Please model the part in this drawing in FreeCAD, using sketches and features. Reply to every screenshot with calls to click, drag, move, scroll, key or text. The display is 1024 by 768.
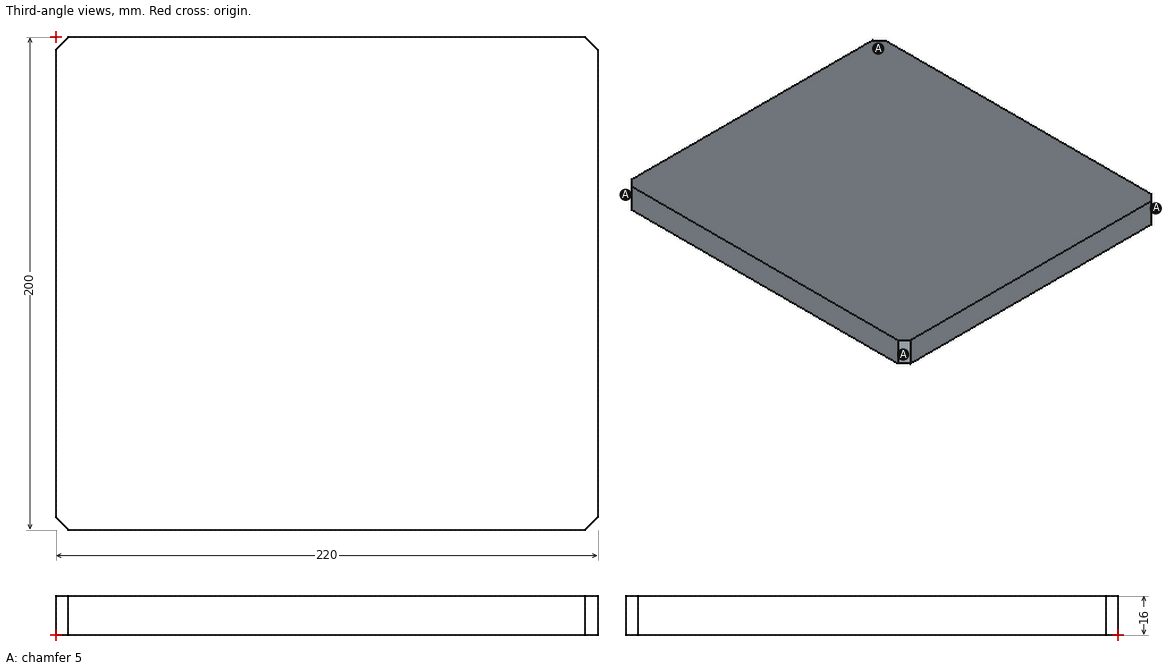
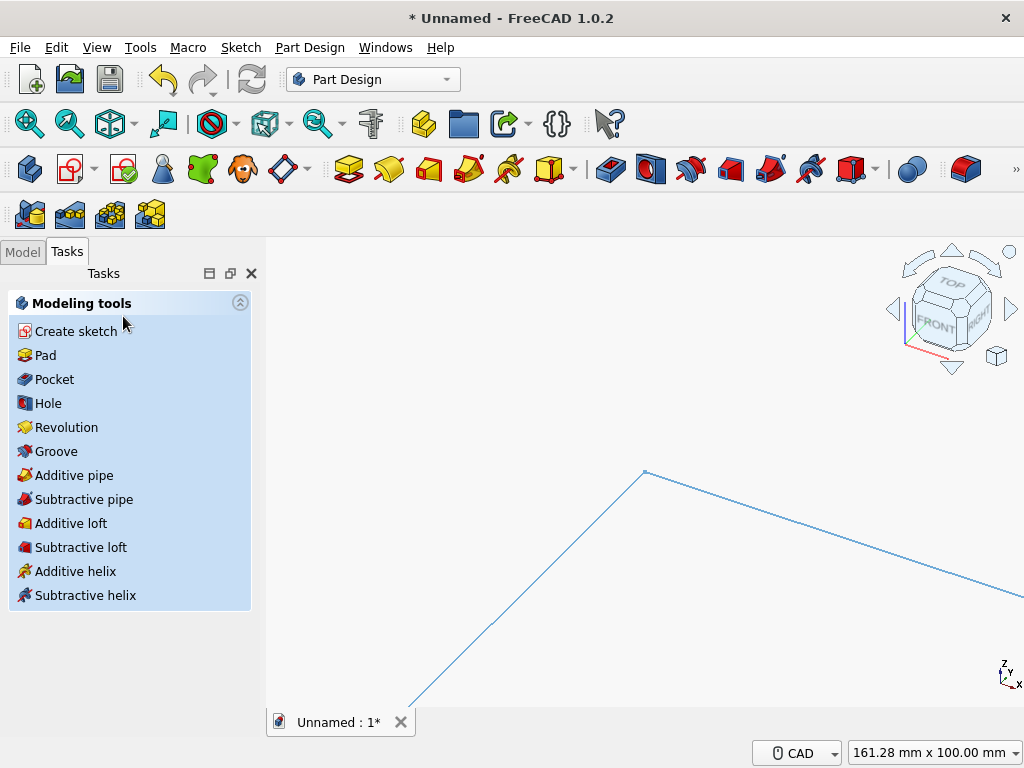
click(350, 170)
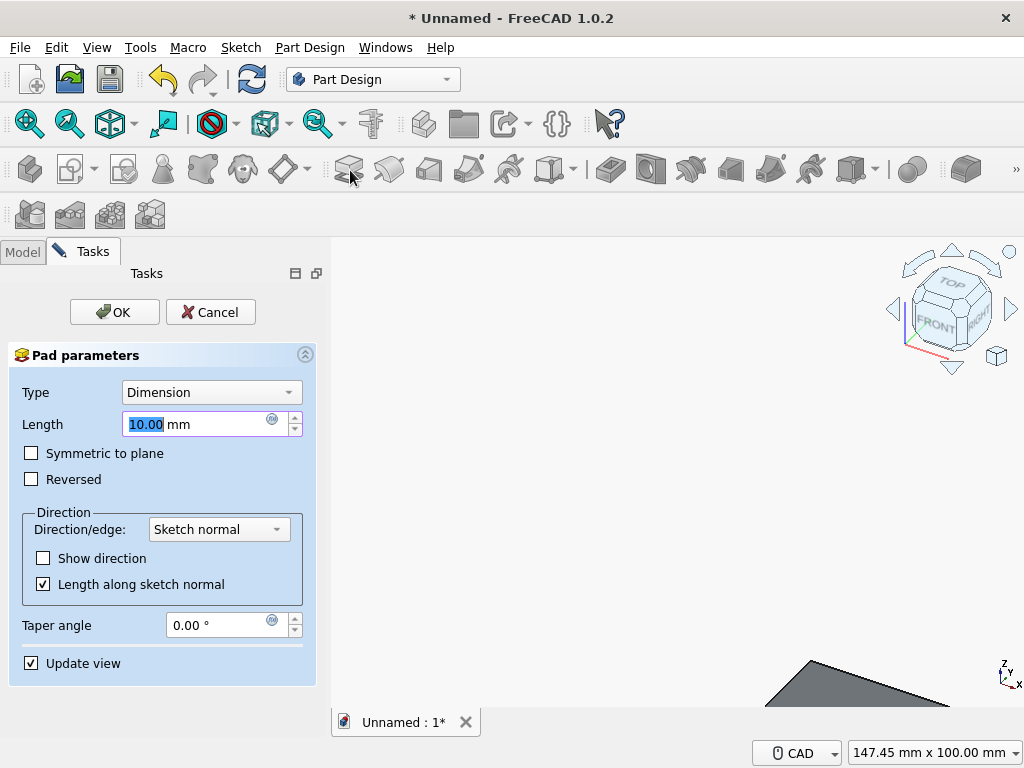
text(16)
key(Tab)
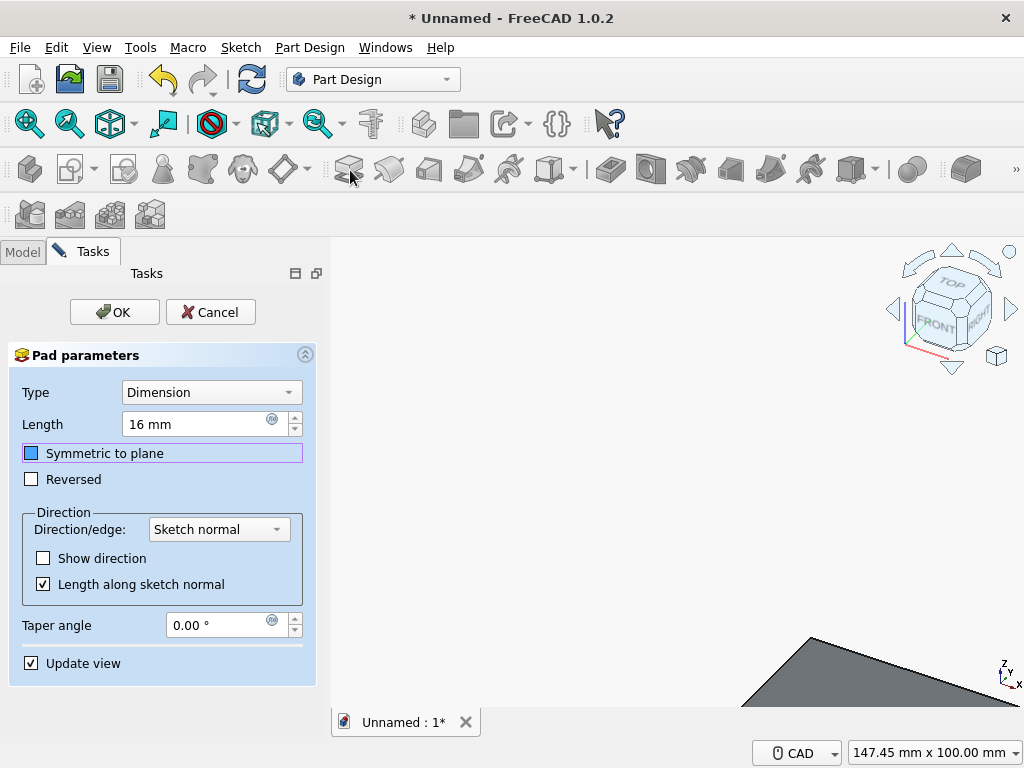
click(115, 312)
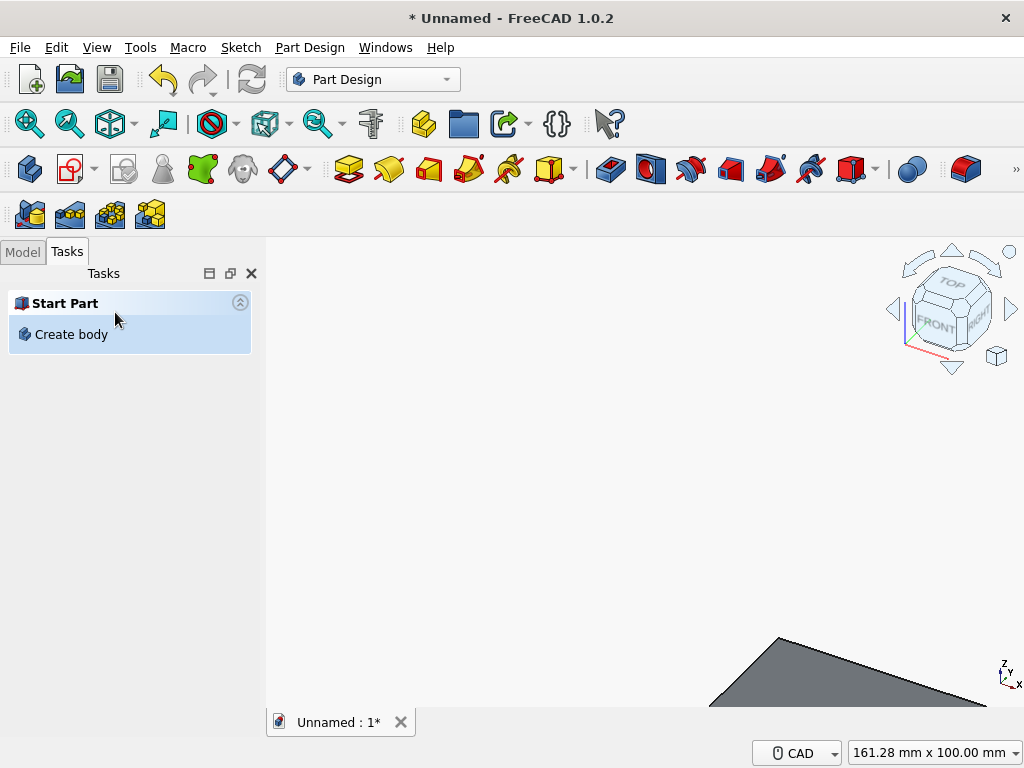
click(30, 124)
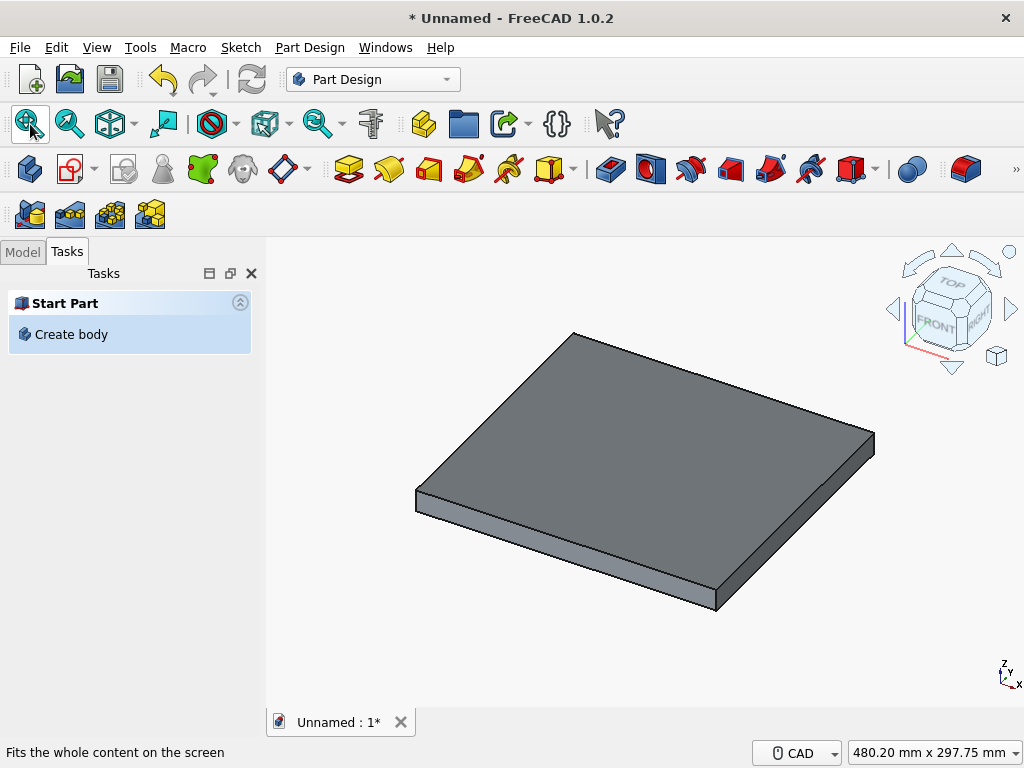
click(716, 599)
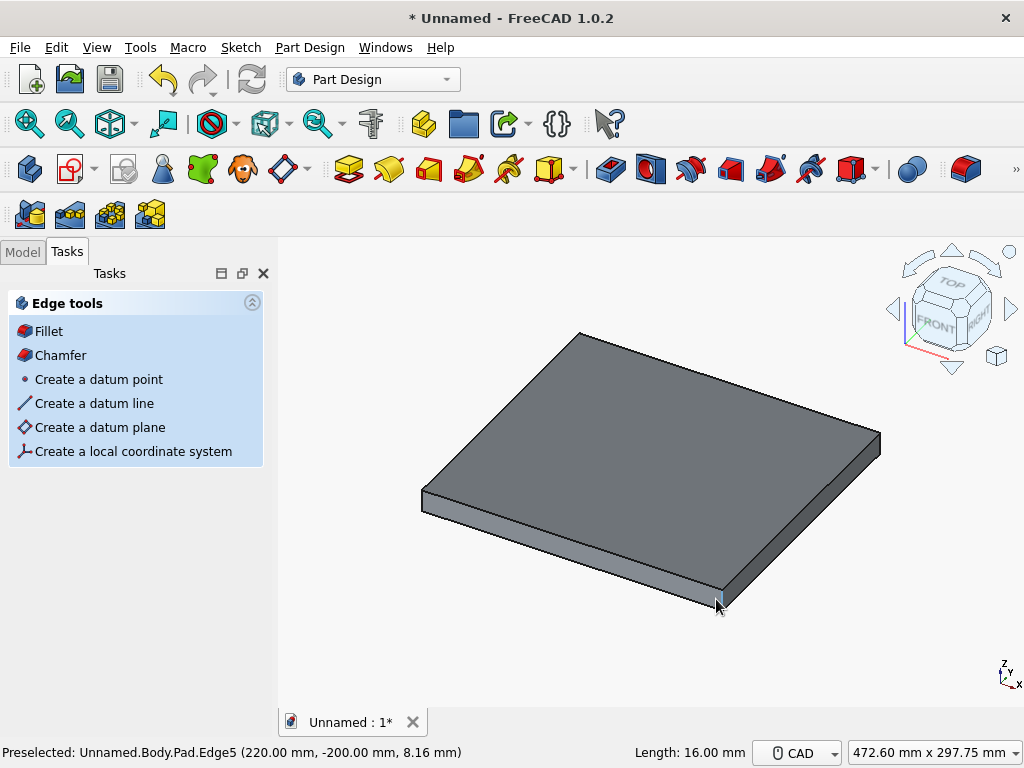
key(0)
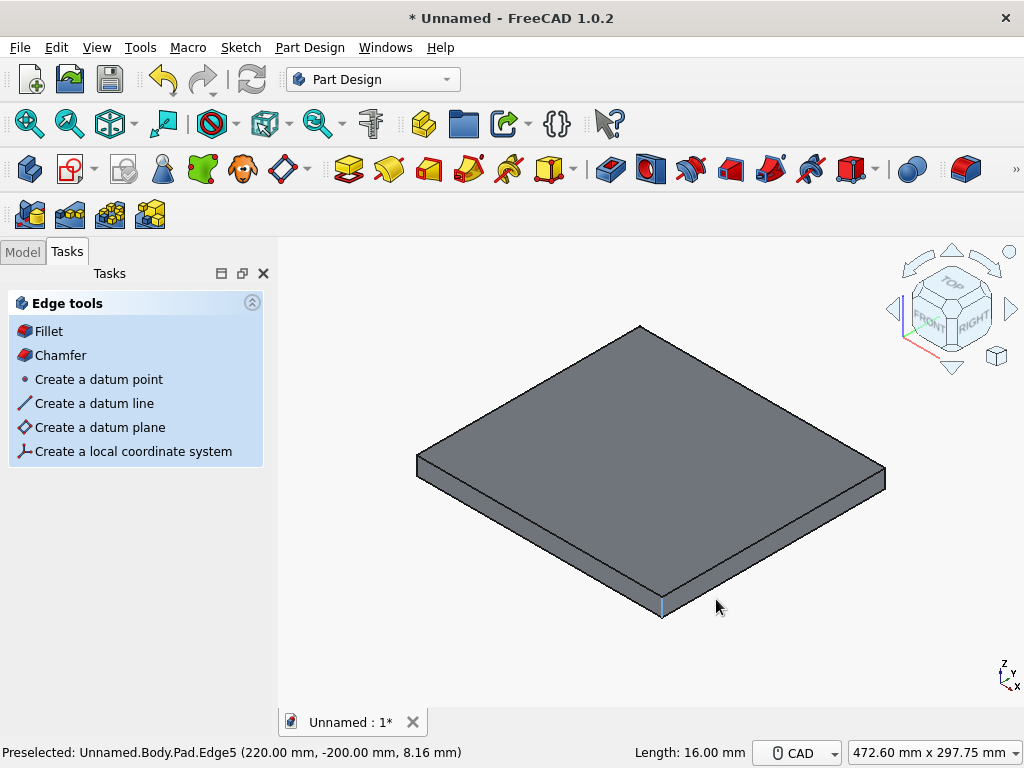
key(2)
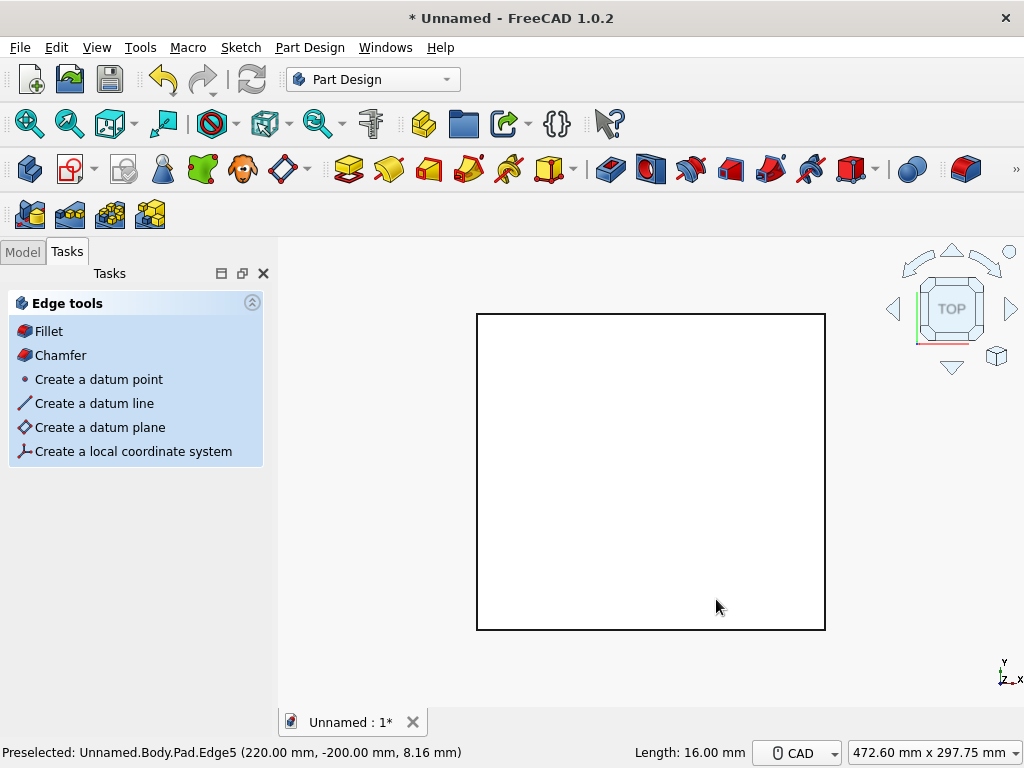
key(1)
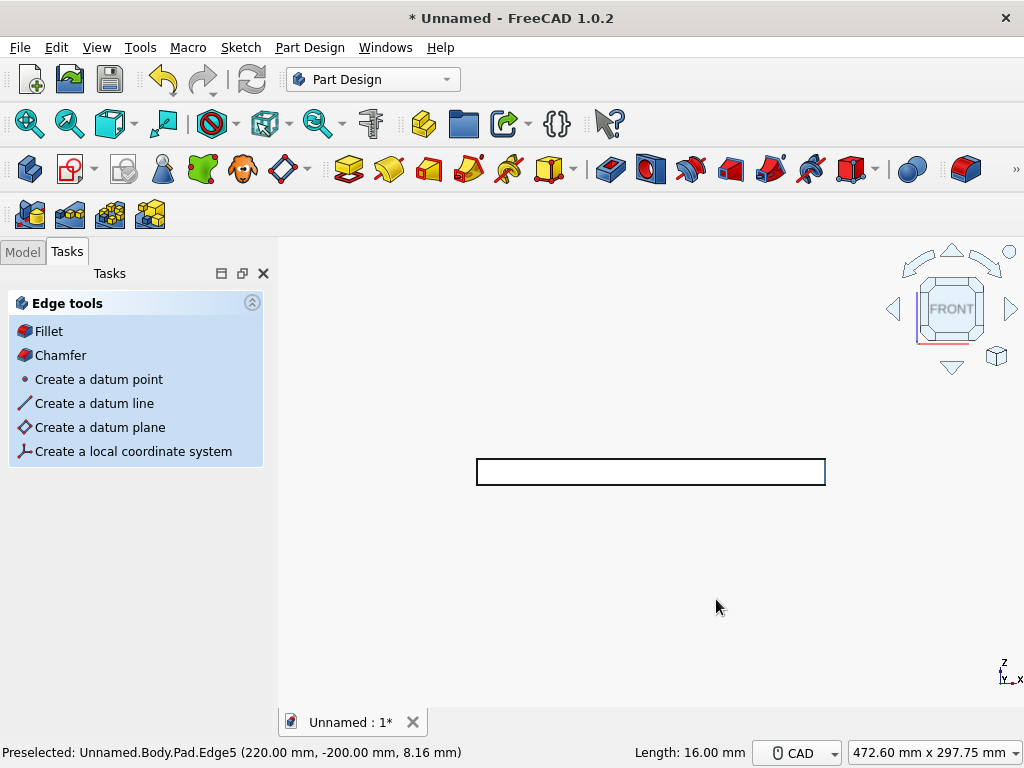
click(477, 471, ctrl)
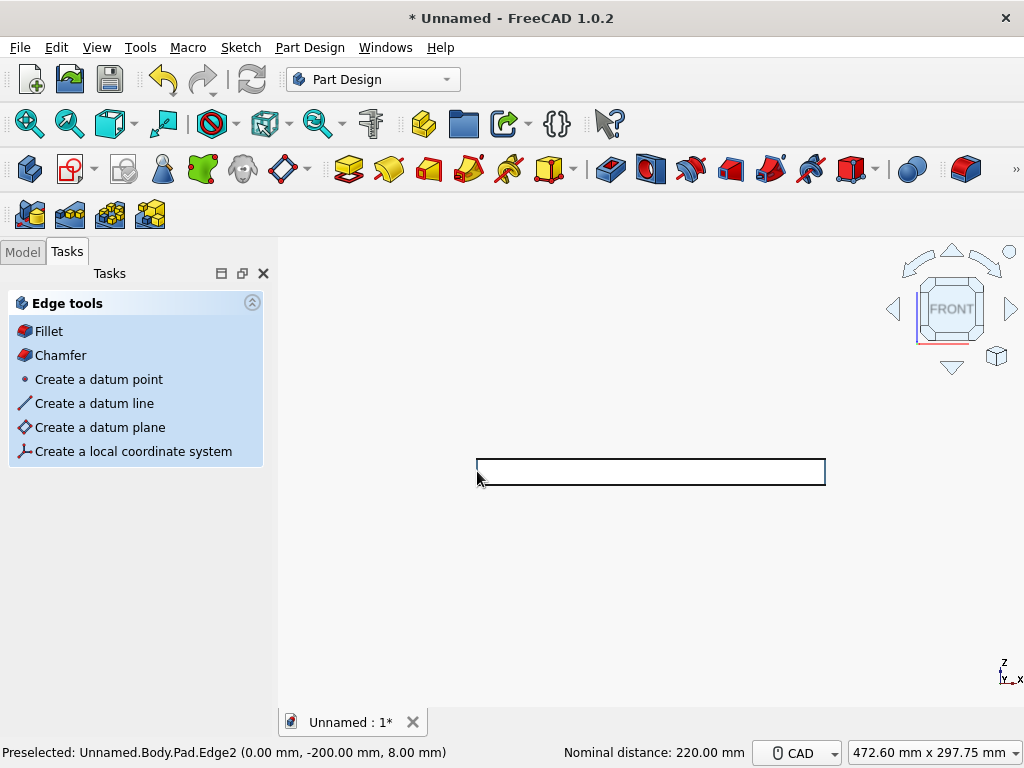
key(3)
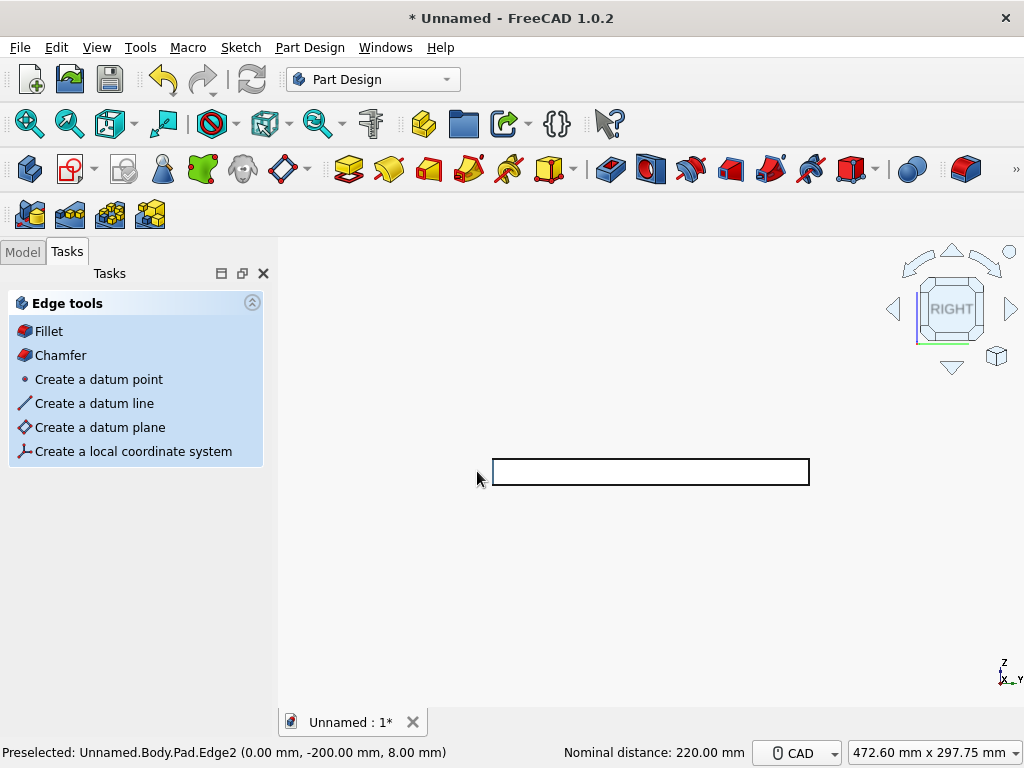
click(30, 124)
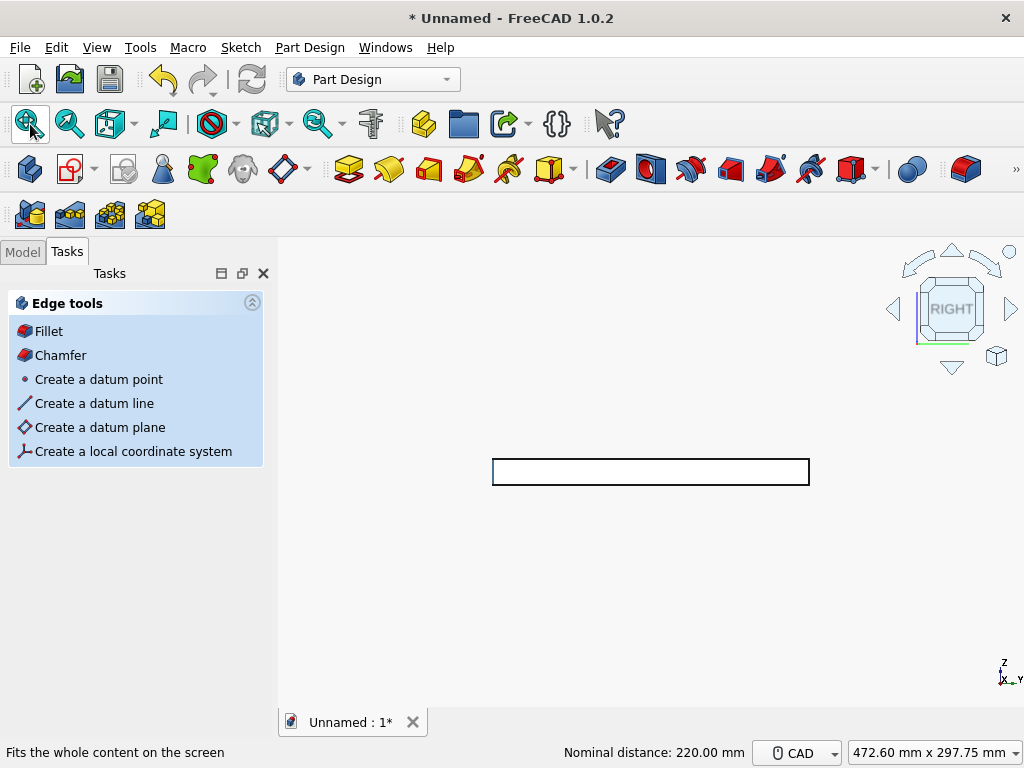
click(809, 471, ctrl)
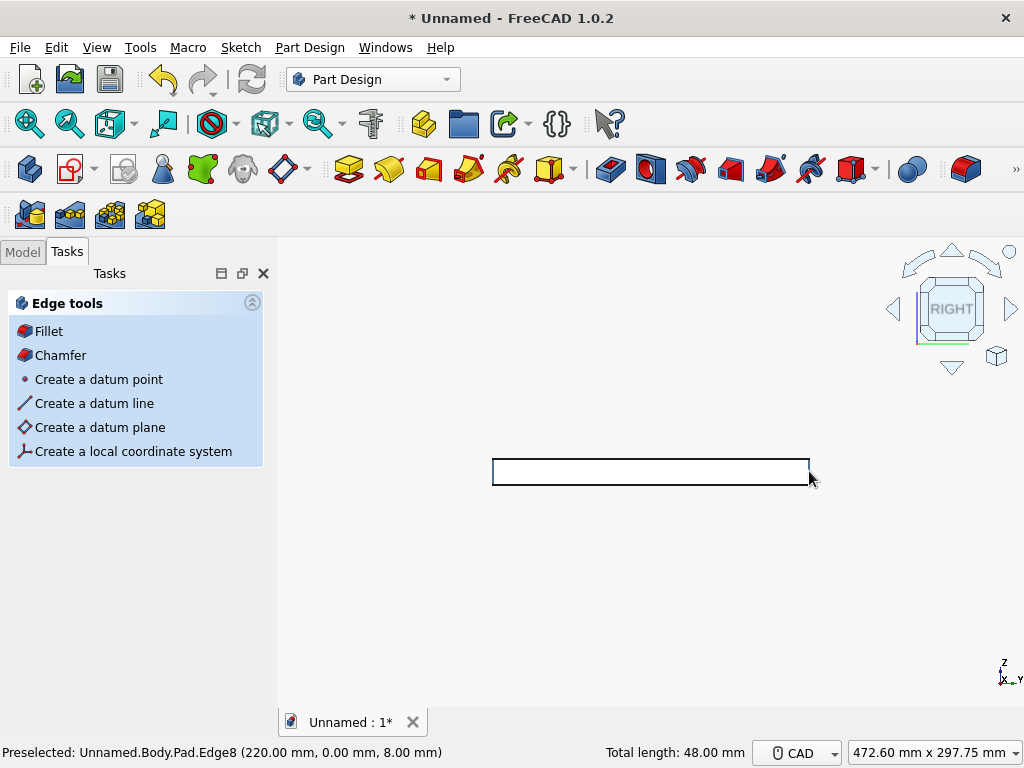
key(5)